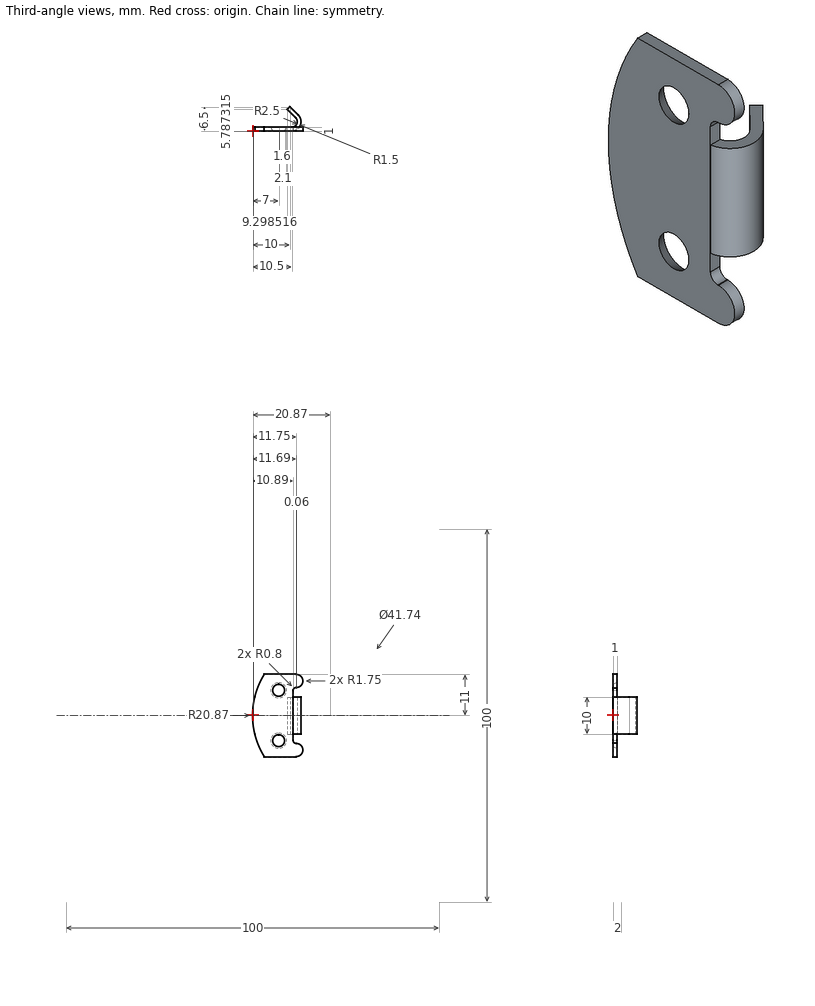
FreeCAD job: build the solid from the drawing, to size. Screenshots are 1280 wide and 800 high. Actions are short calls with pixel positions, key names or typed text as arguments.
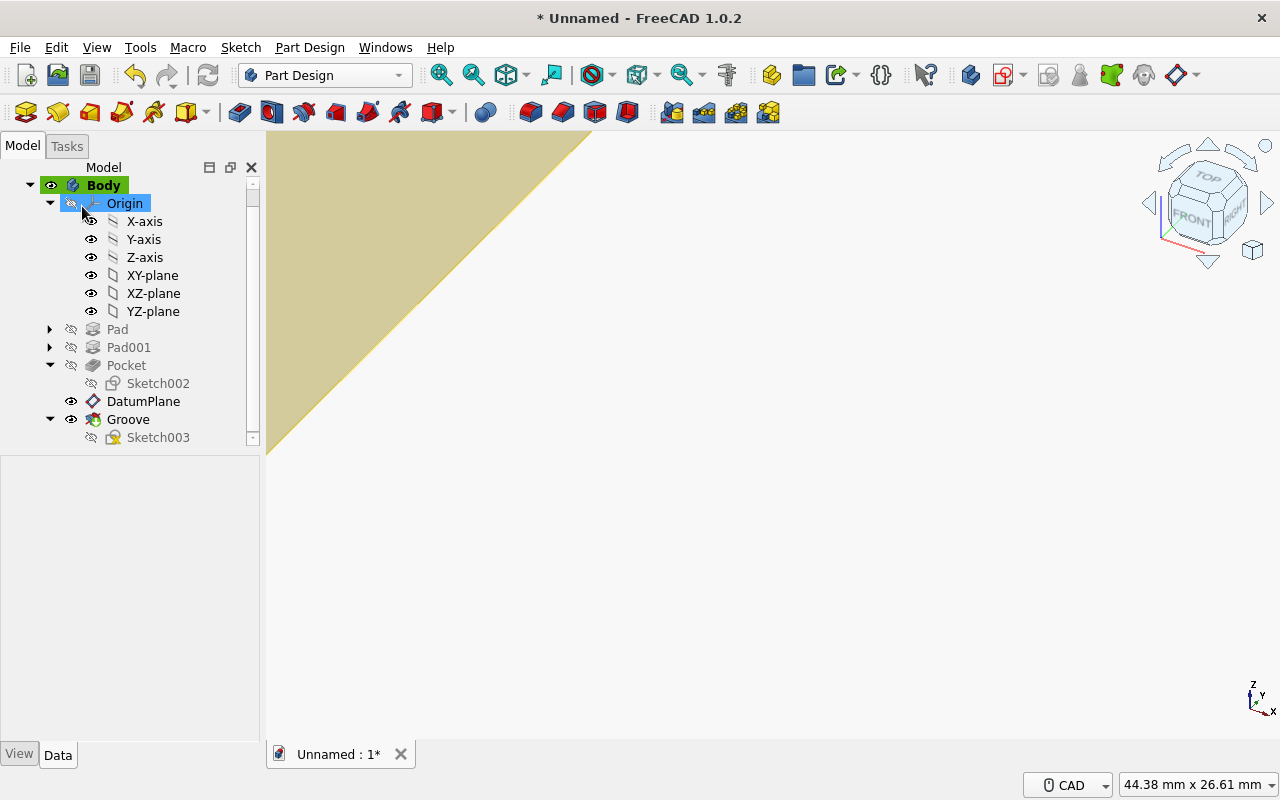
click(116, 401)
key(space)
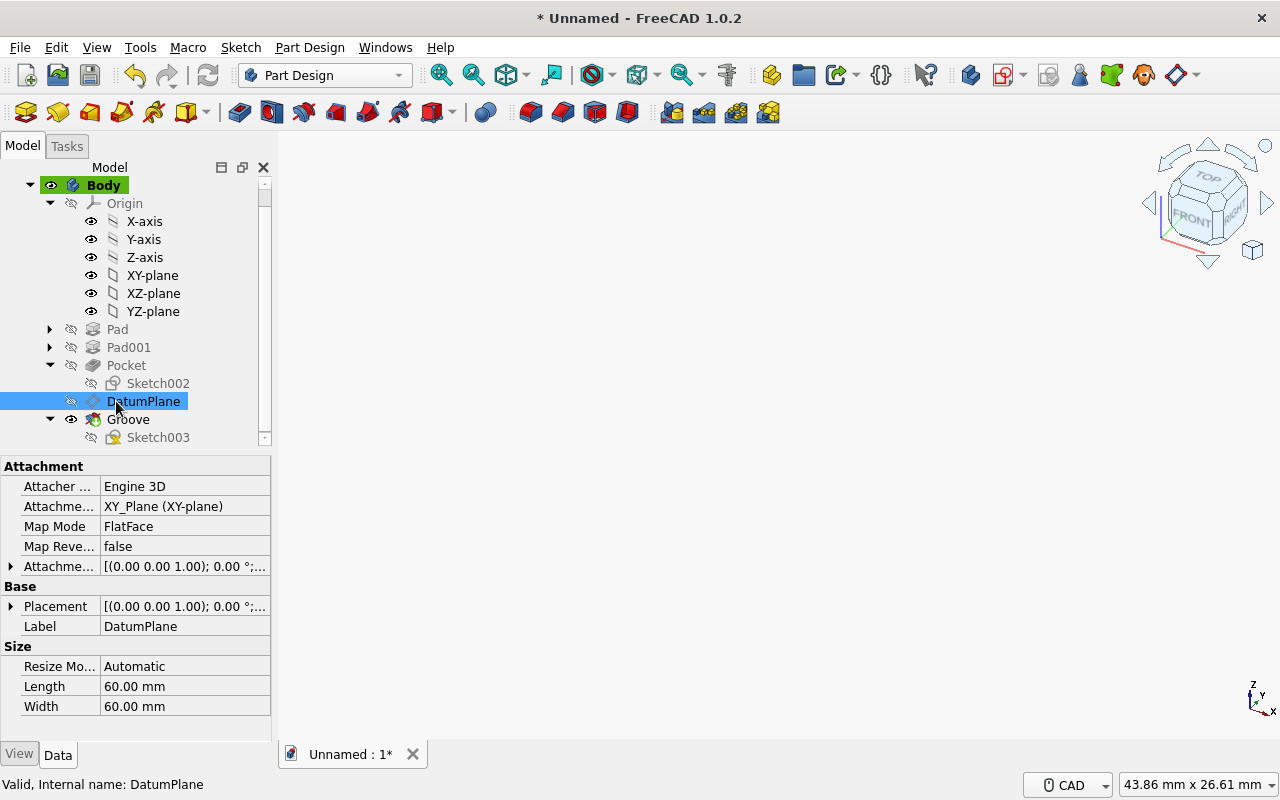
click(442, 76)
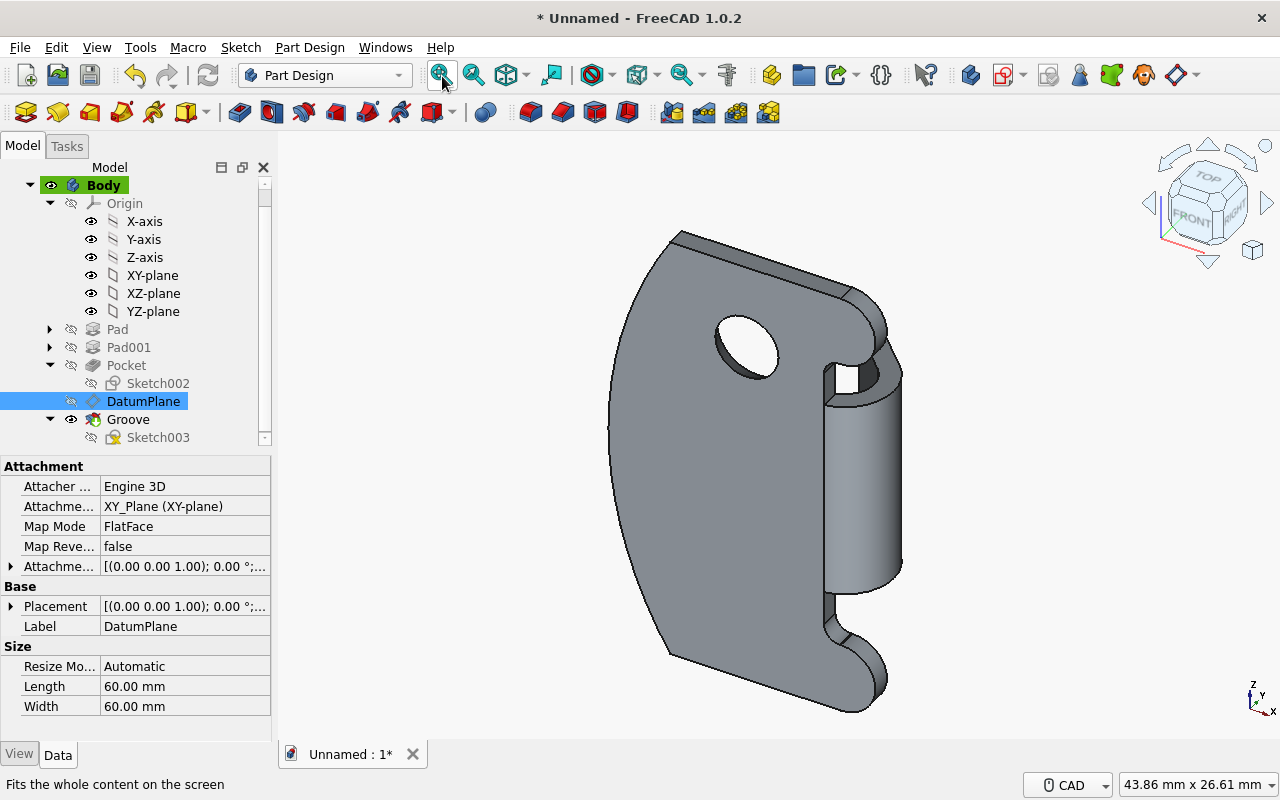
click(136, 275)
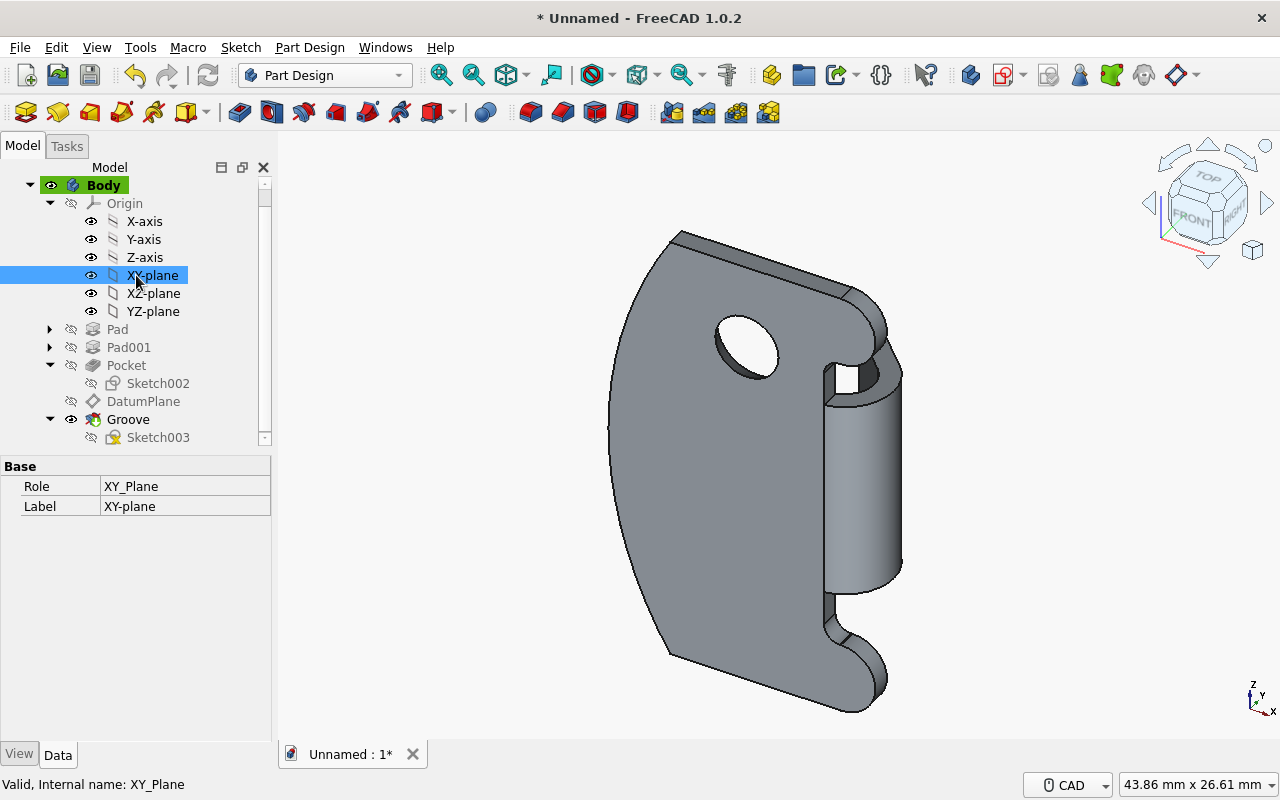
click(1176, 76)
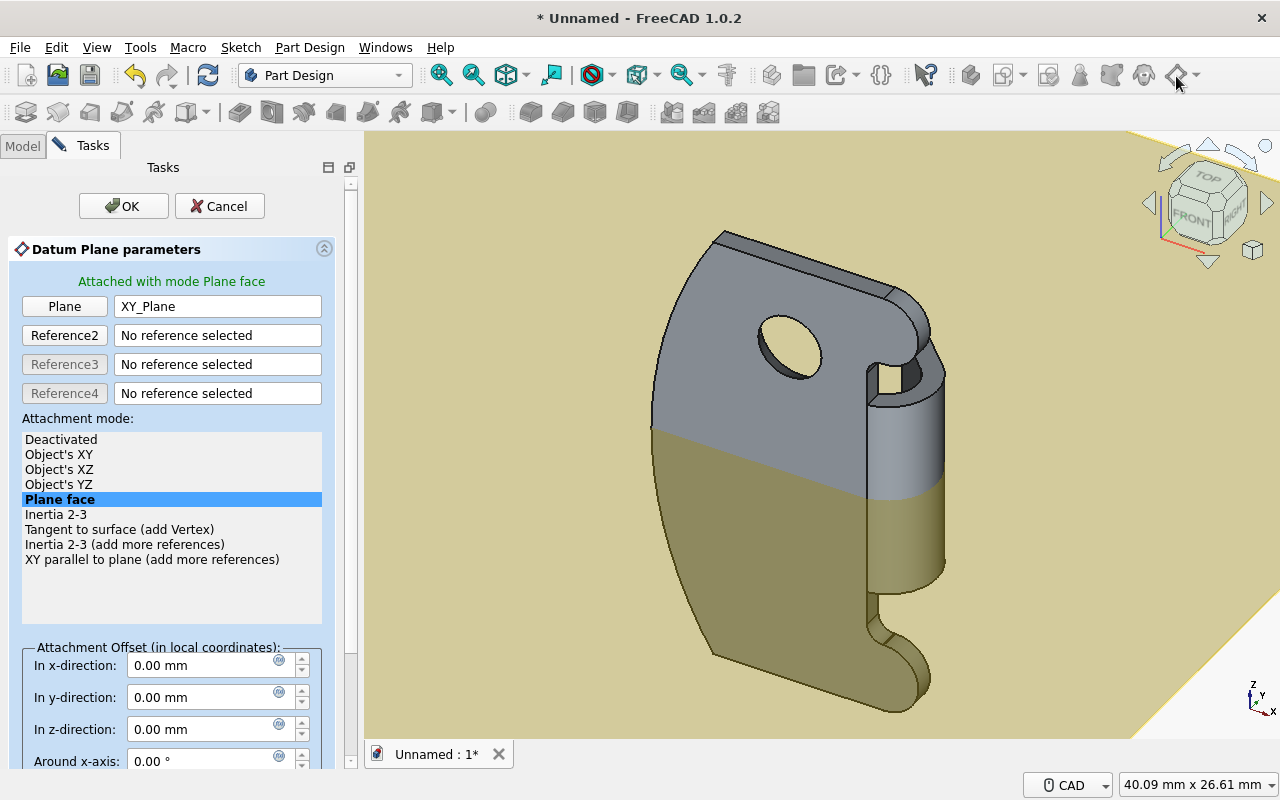
triple_click(210, 729)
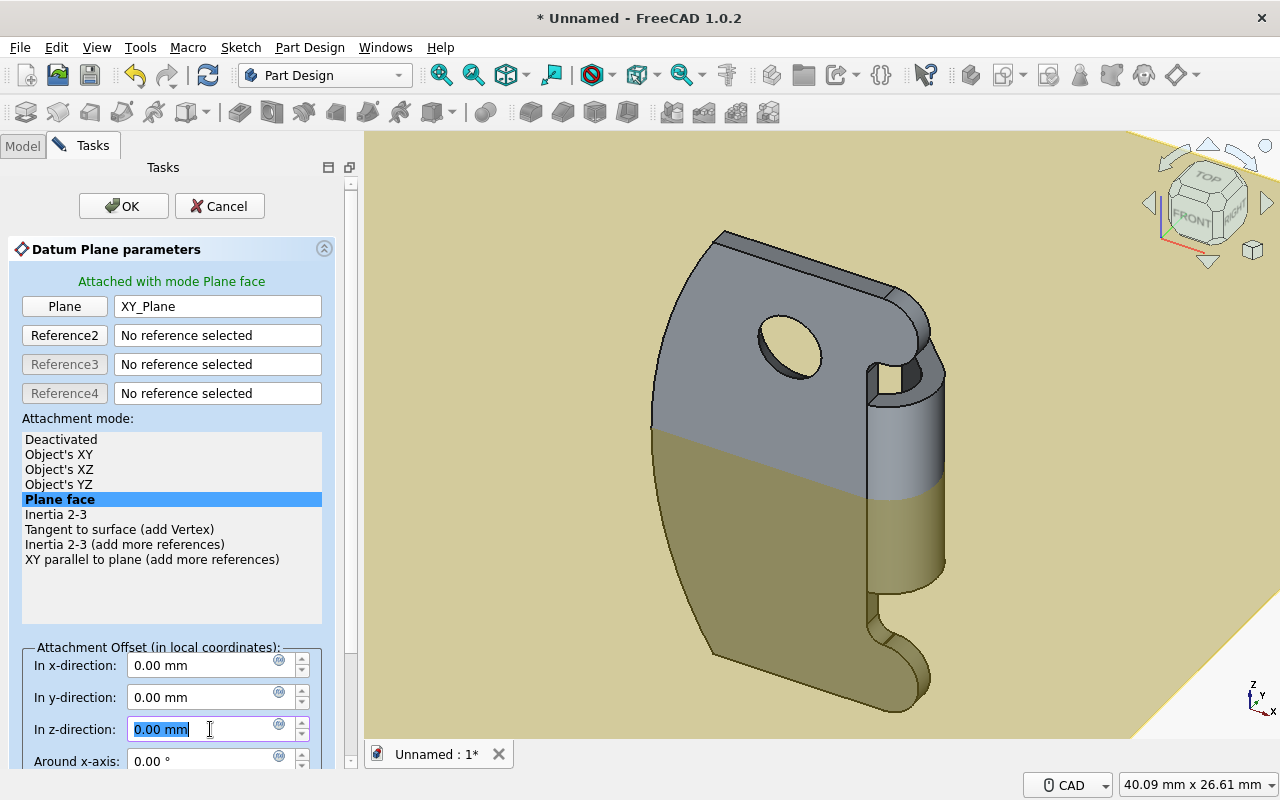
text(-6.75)
key(Tab)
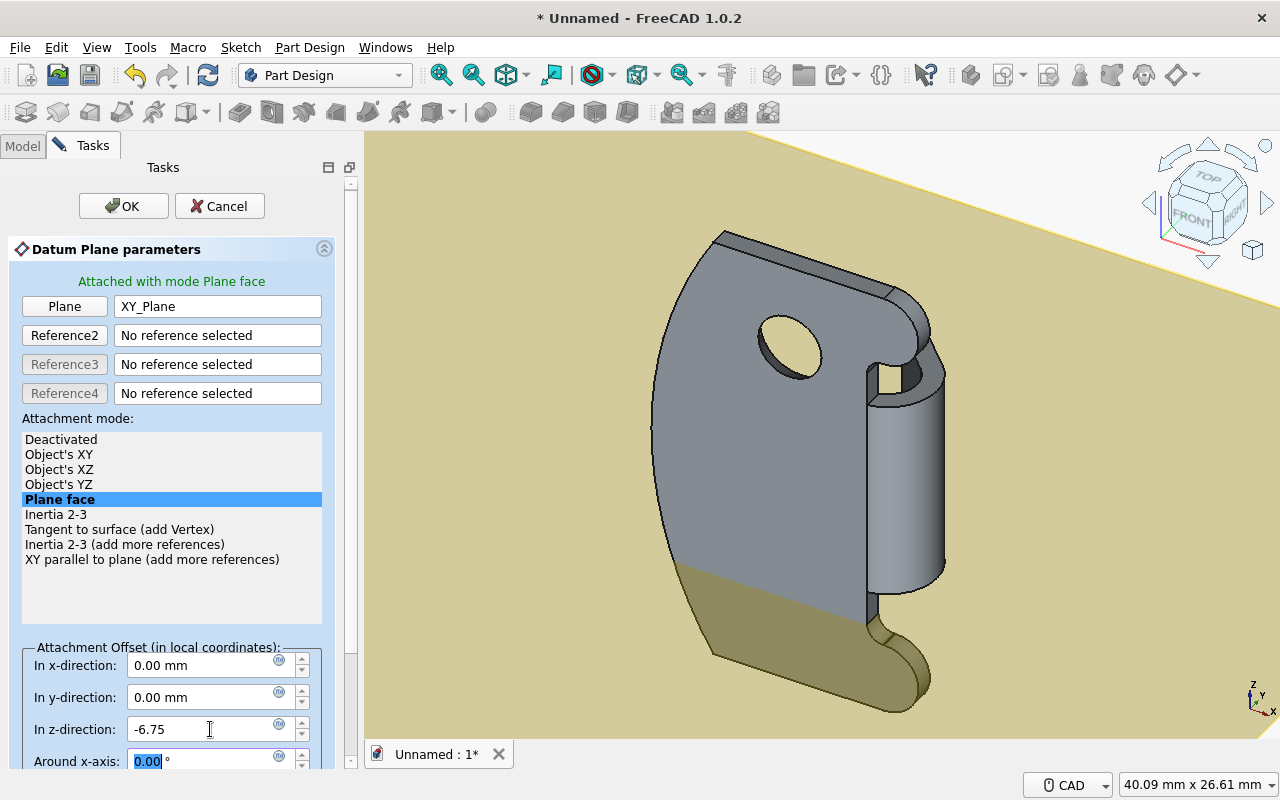
click(124, 206)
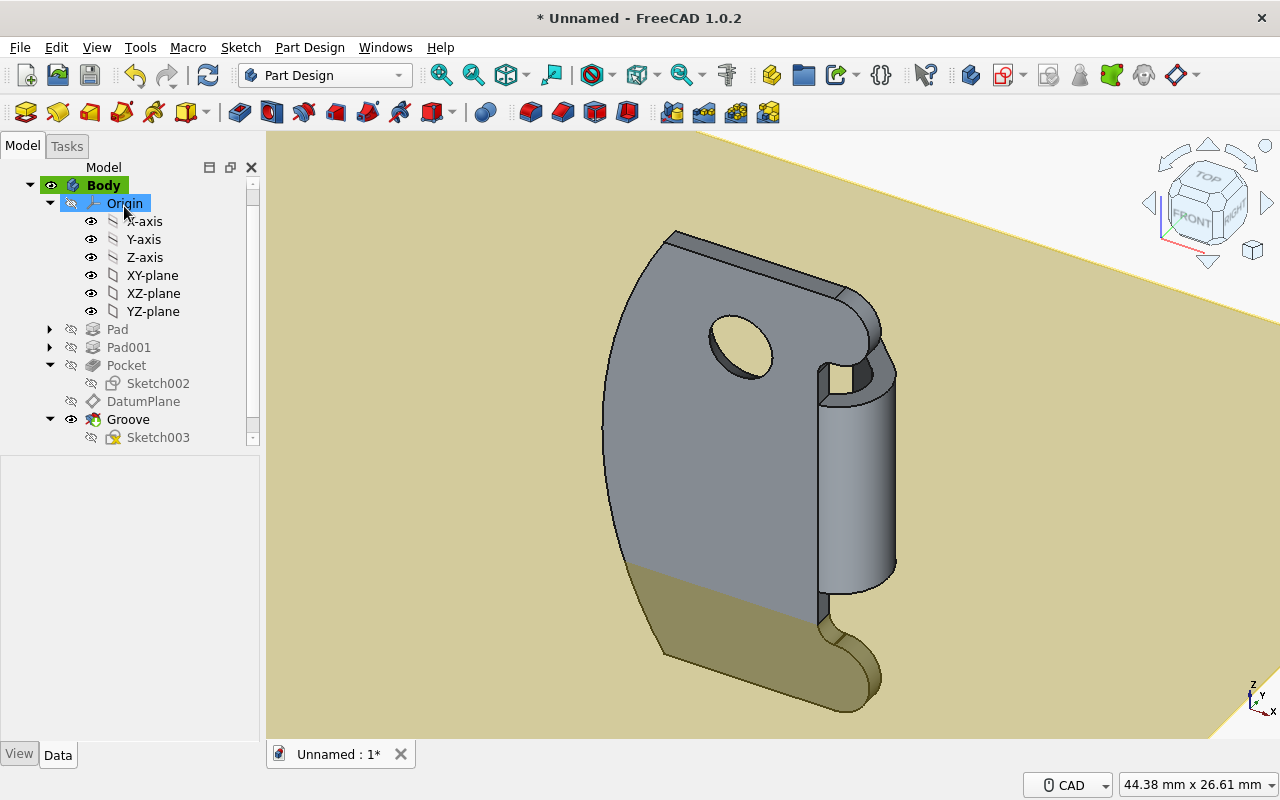
scroll(120, 307, down, 3)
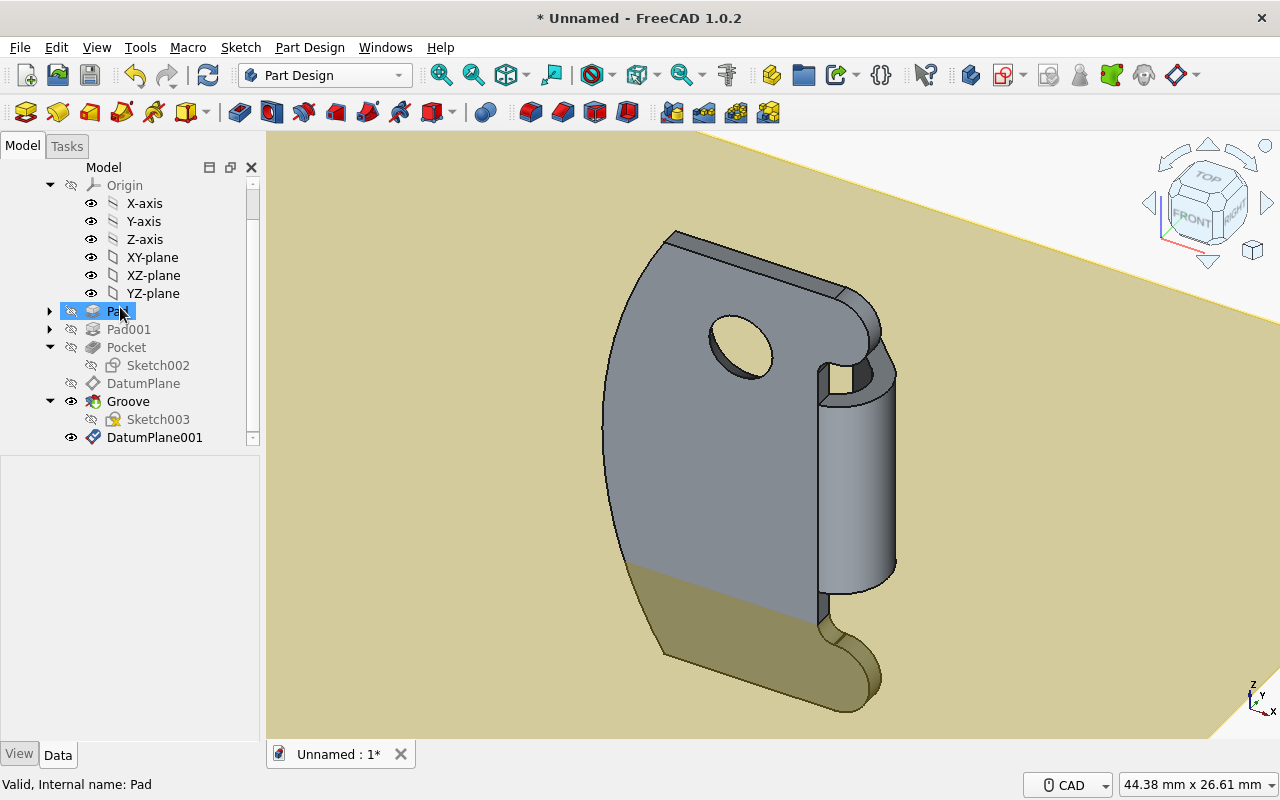
click(116, 437)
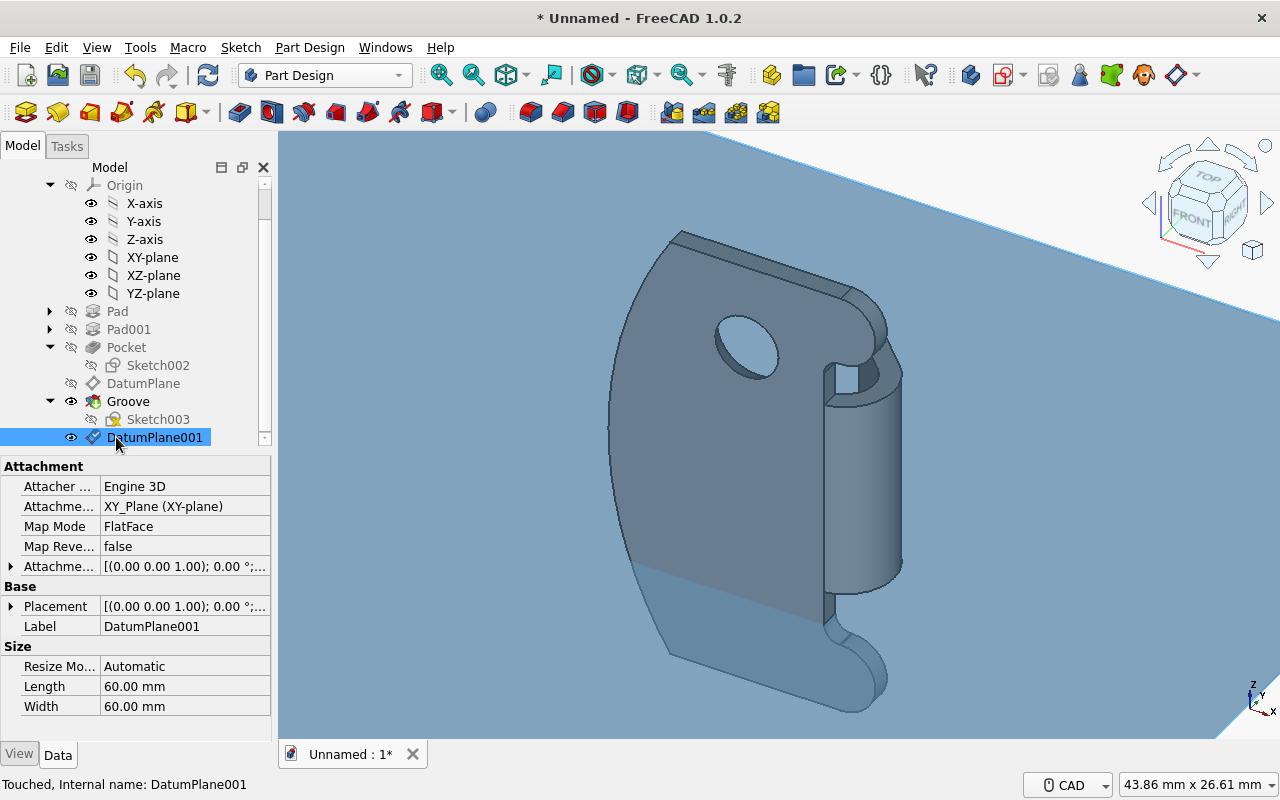
click(1004, 76)